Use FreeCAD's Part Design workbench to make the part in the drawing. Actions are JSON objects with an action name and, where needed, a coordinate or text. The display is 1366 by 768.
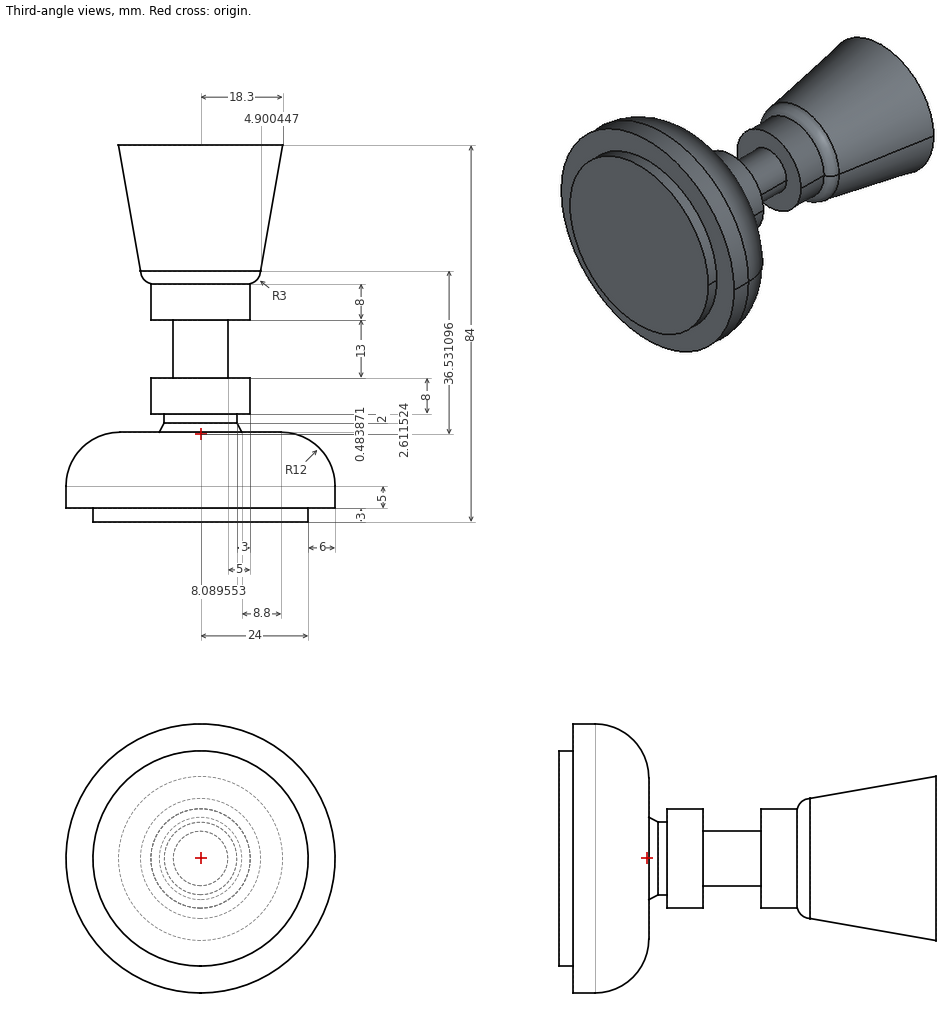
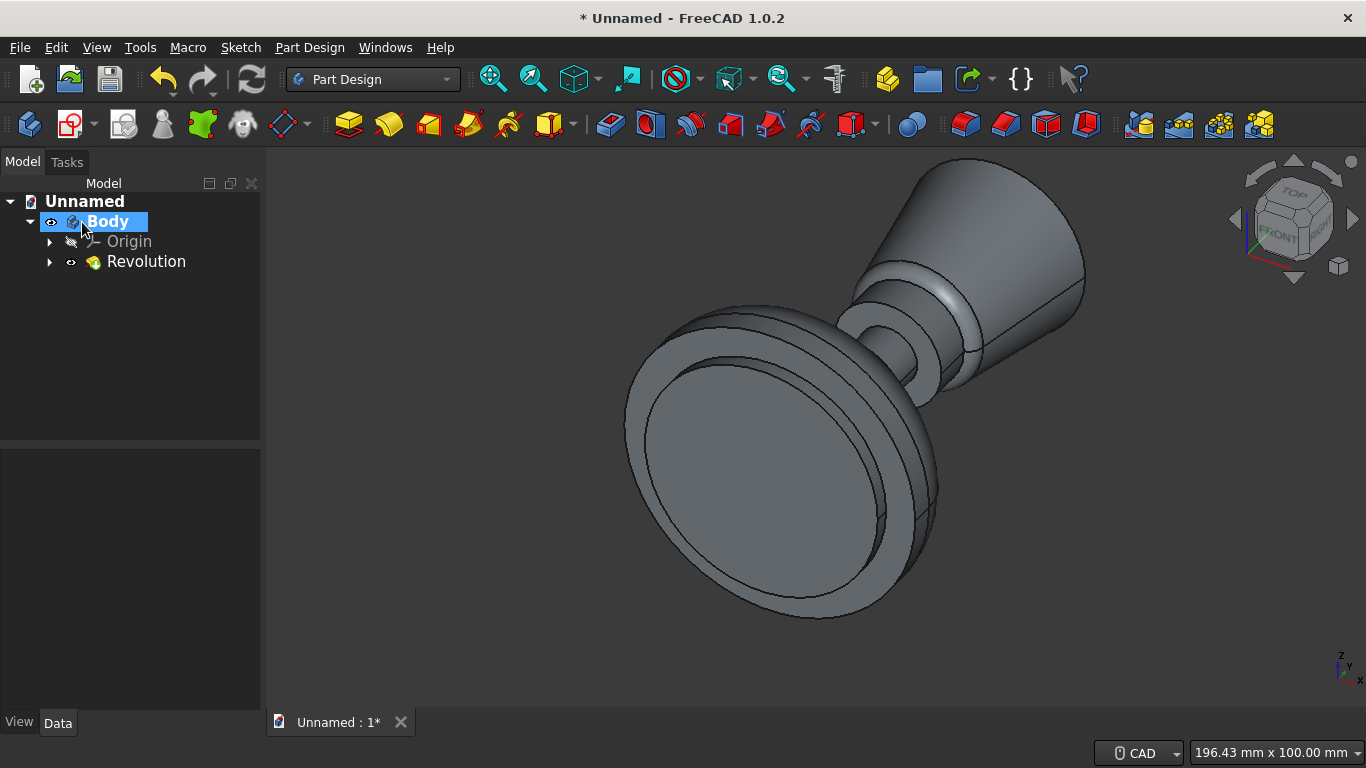
{"action": "key", "text": "0"}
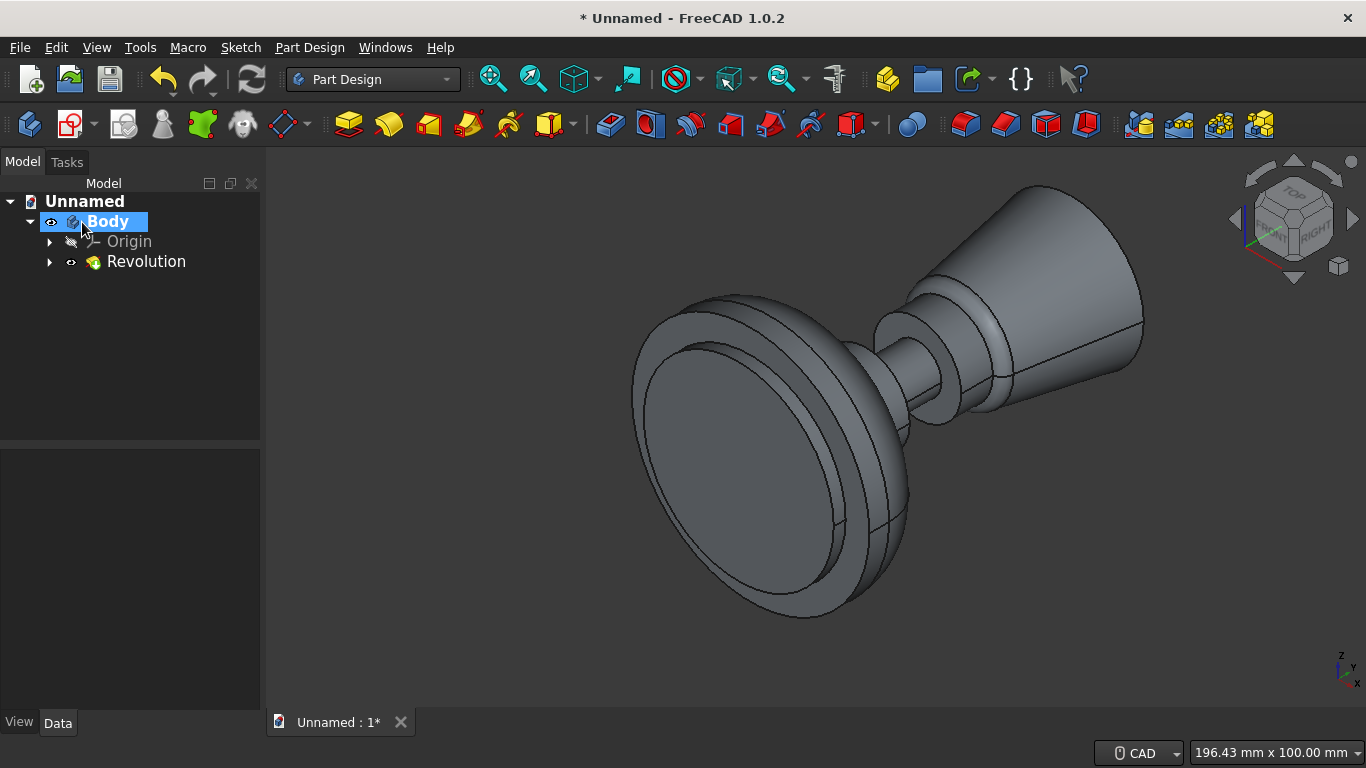
{"action": "left_click", "coordinate": [494, 80]}